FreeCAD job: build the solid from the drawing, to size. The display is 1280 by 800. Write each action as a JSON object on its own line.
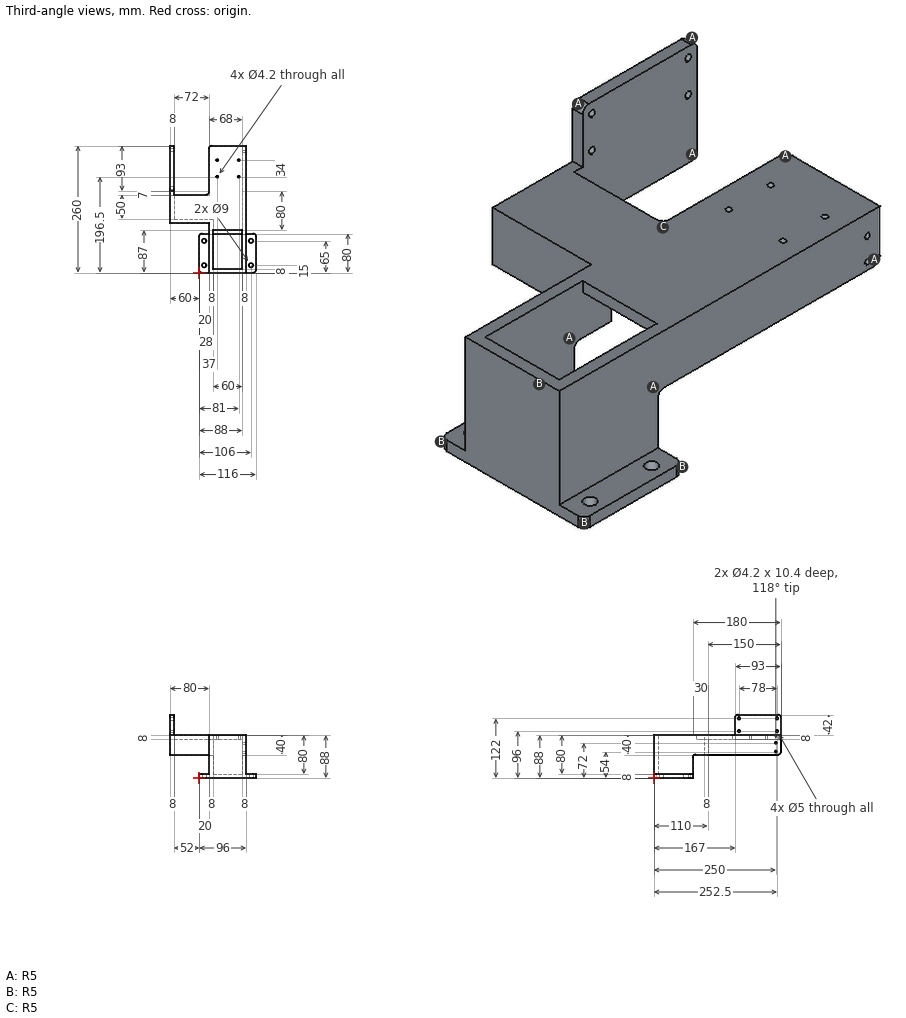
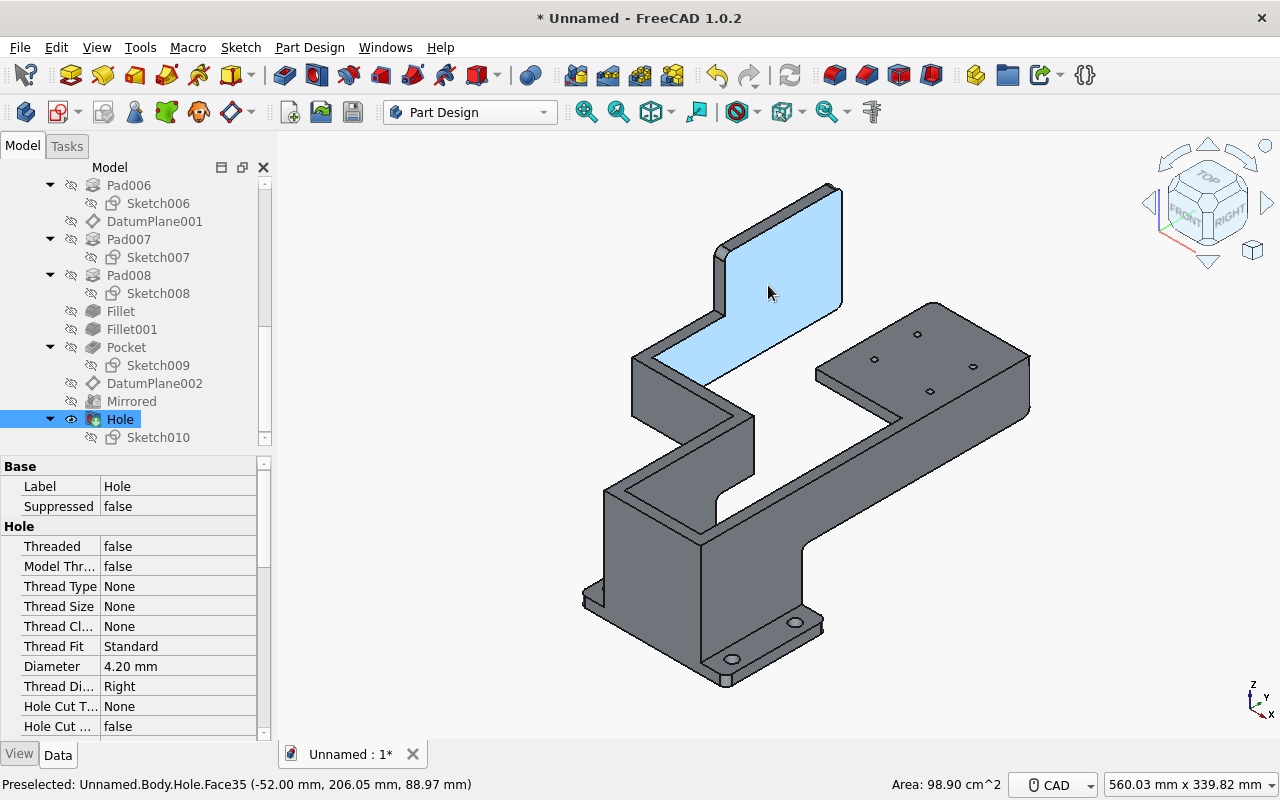
{"action": "left_click", "coordinate": [58, 112]}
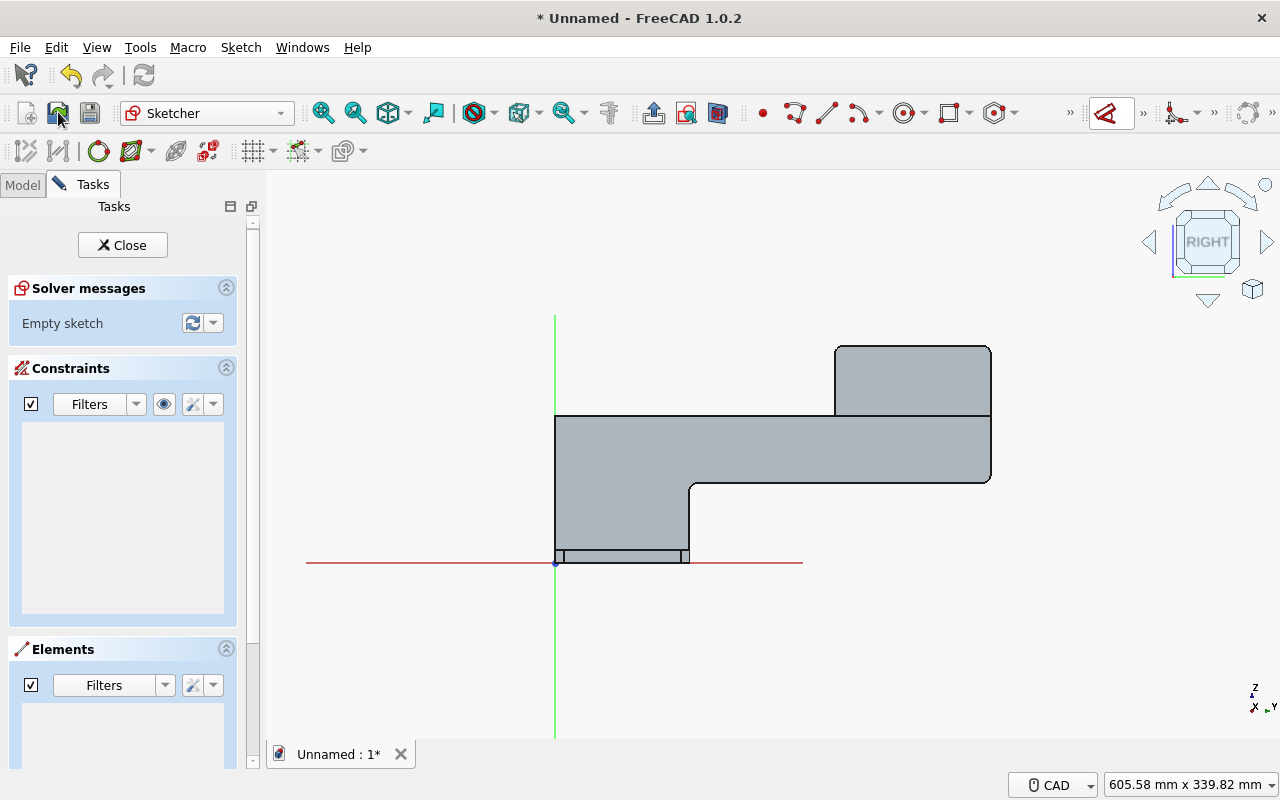
{"action": "left_click", "coordinate": [718, 114]}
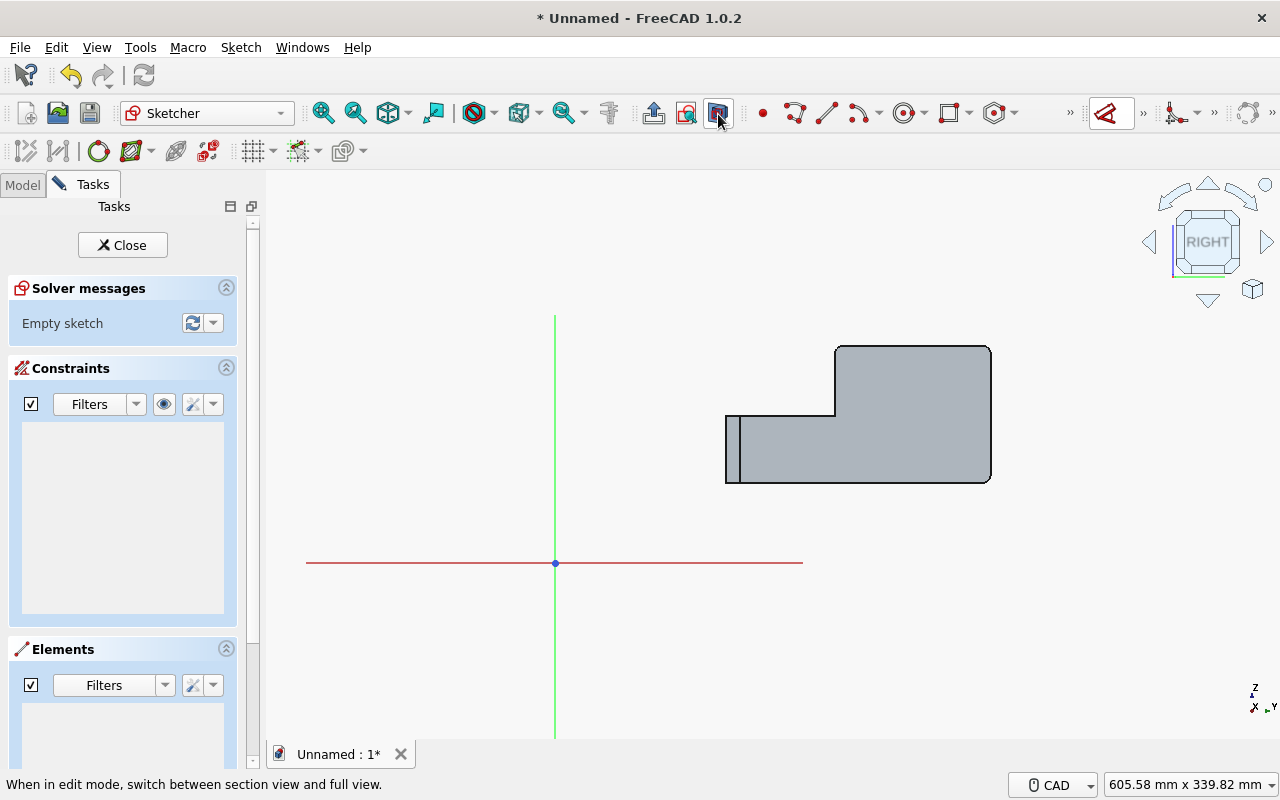
{"action": "scroll", "coordinate": [981, 357], "scroll_direction": "up", "scroll_amount": 7}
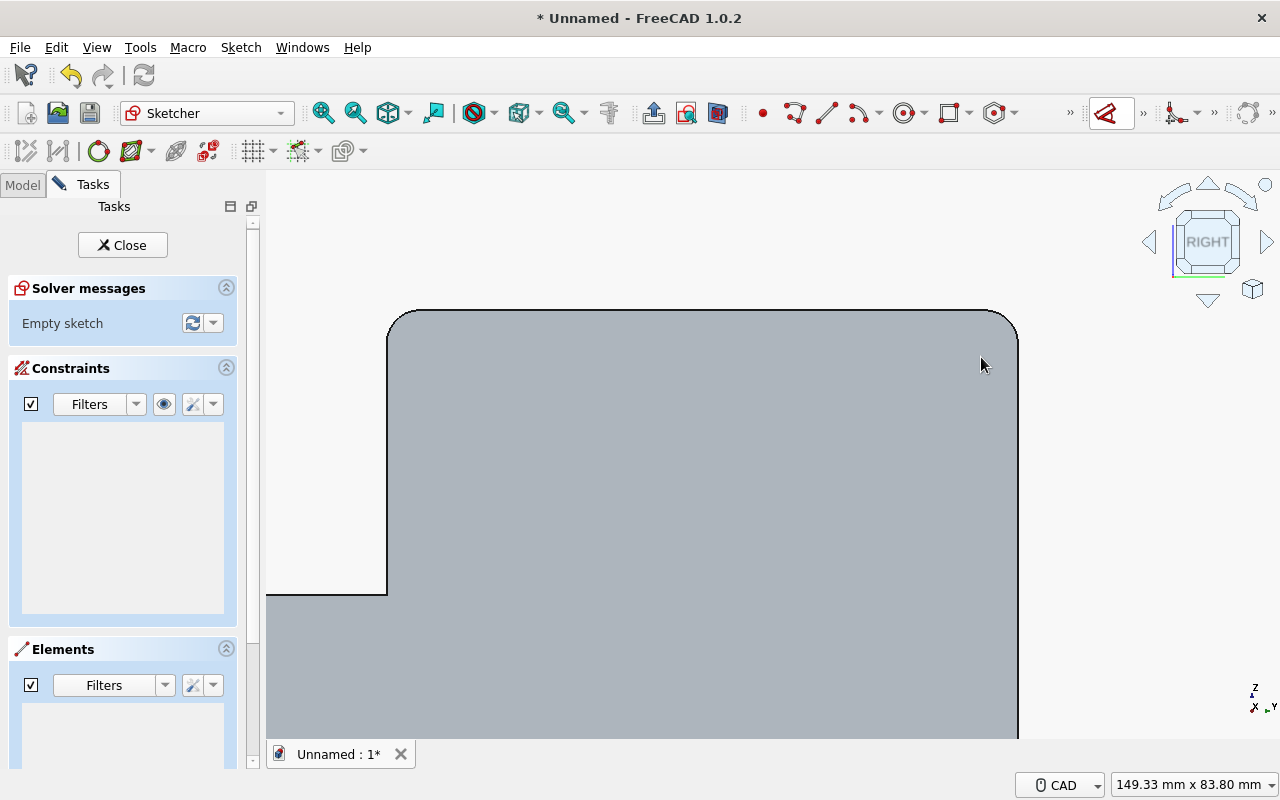
{"action": "left_click", "coordinate": [904, 114]}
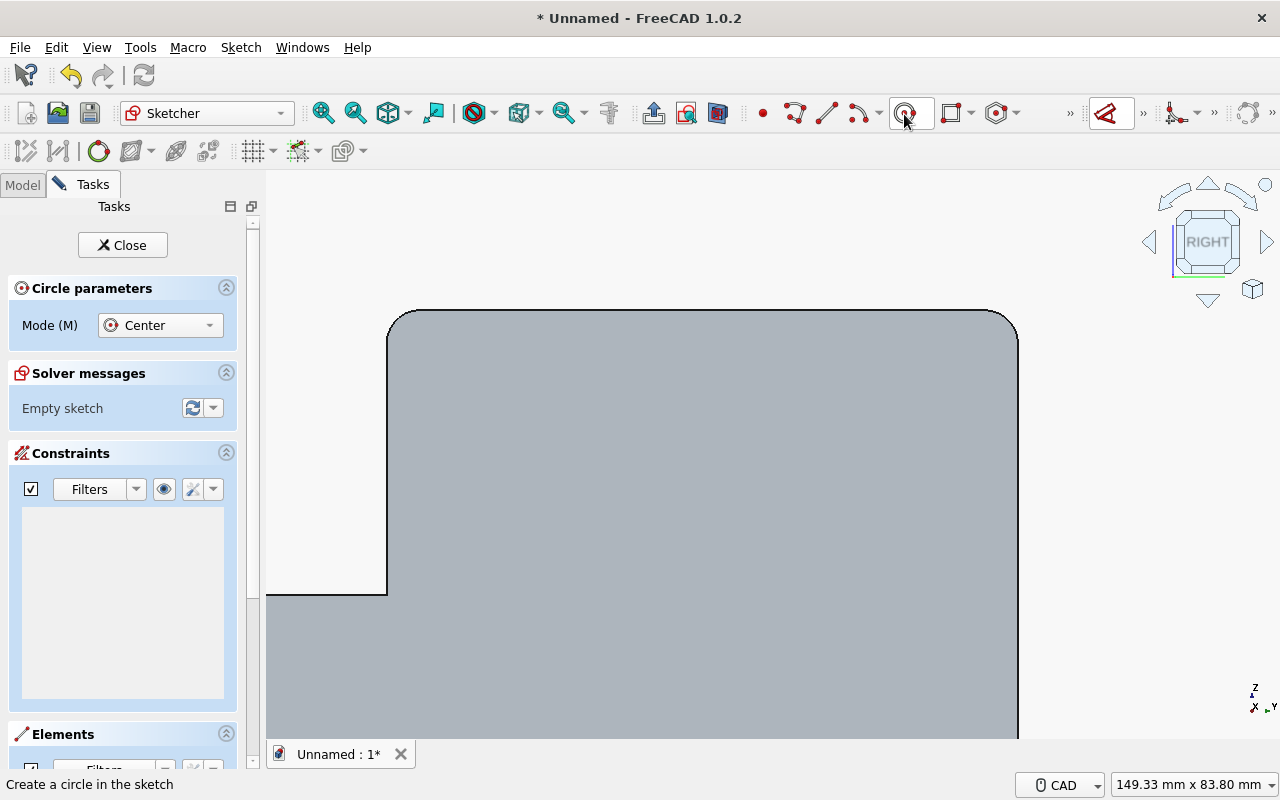
{"action": "scroll", "coordinate": [967, 541], "scroll_direction": "up", "scroll_amount": 2}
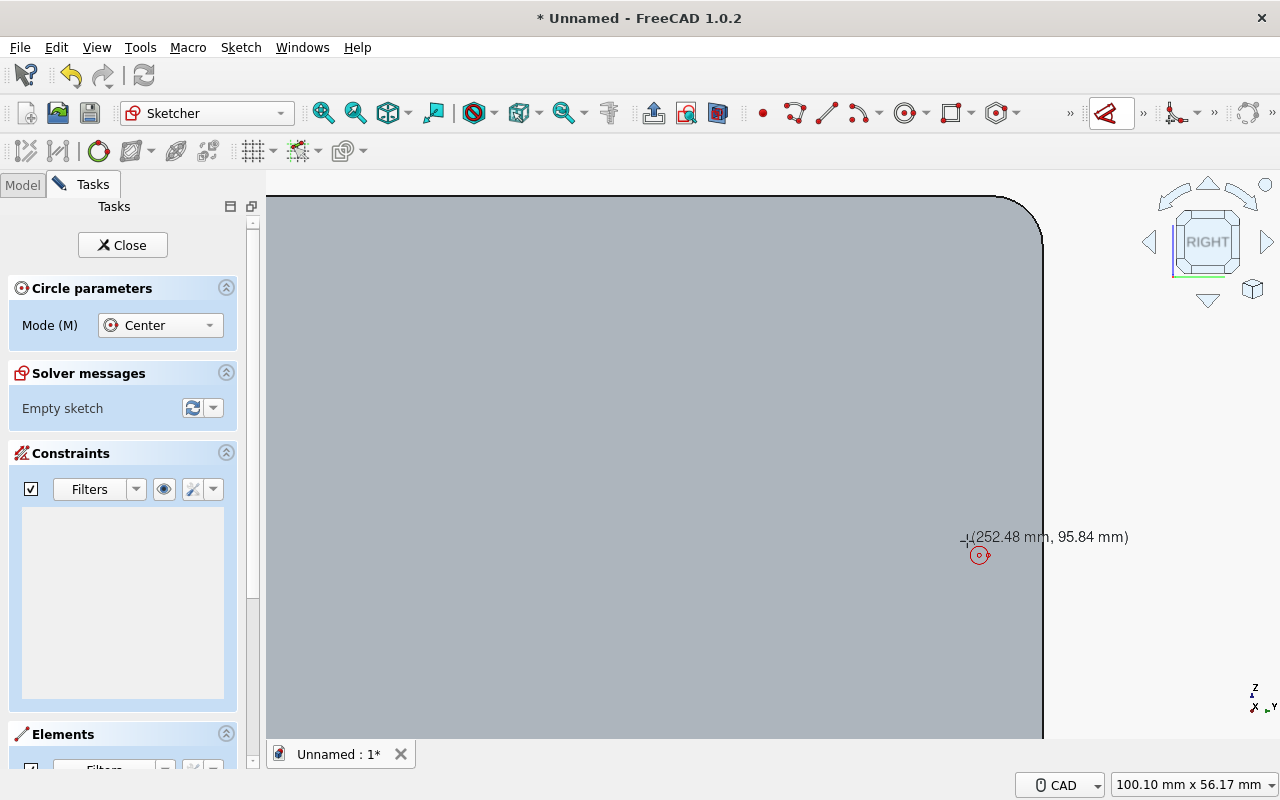
{"action": "left_click", "coordinate": [967, 541]}
{"action": "left_click", "coordinate": [985, 523]}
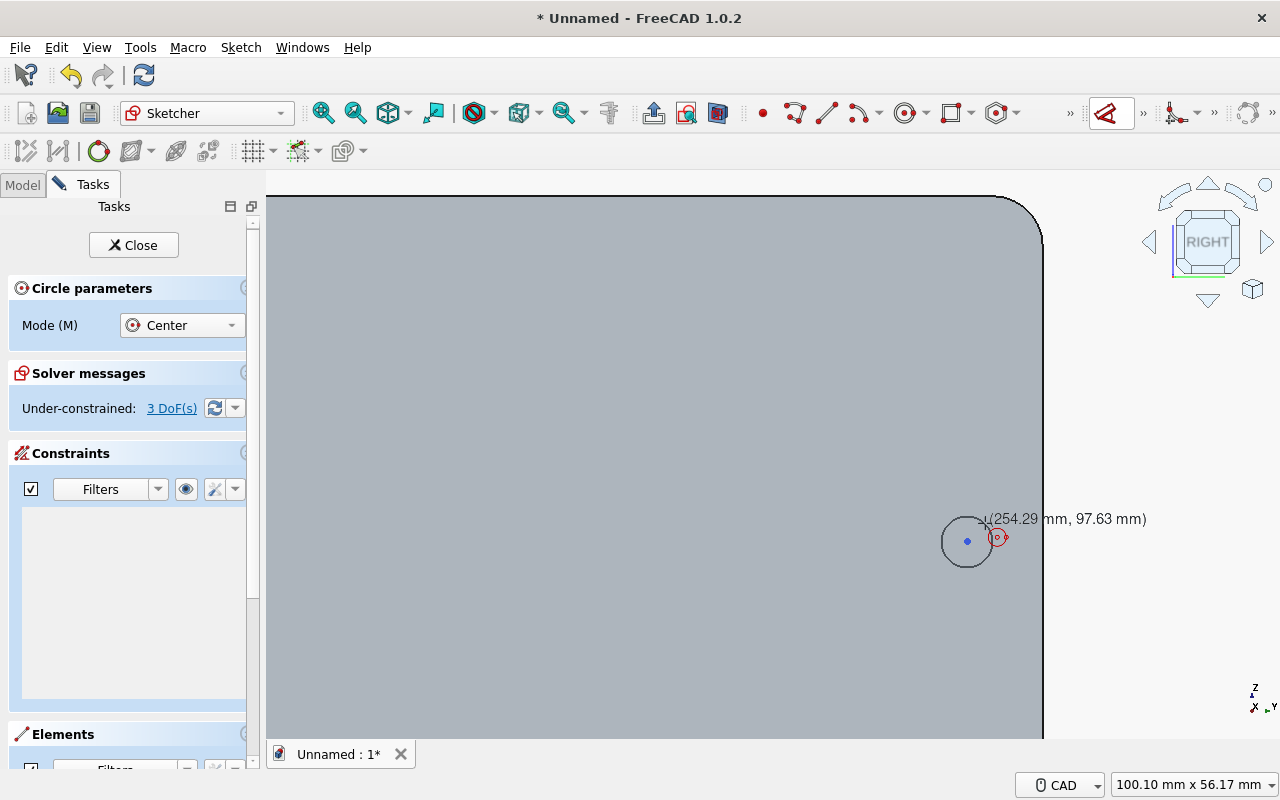
{"action": "left_click", "coordinate": [967, 277]}
{"action": "left_click", "coordinate": [985, 259]}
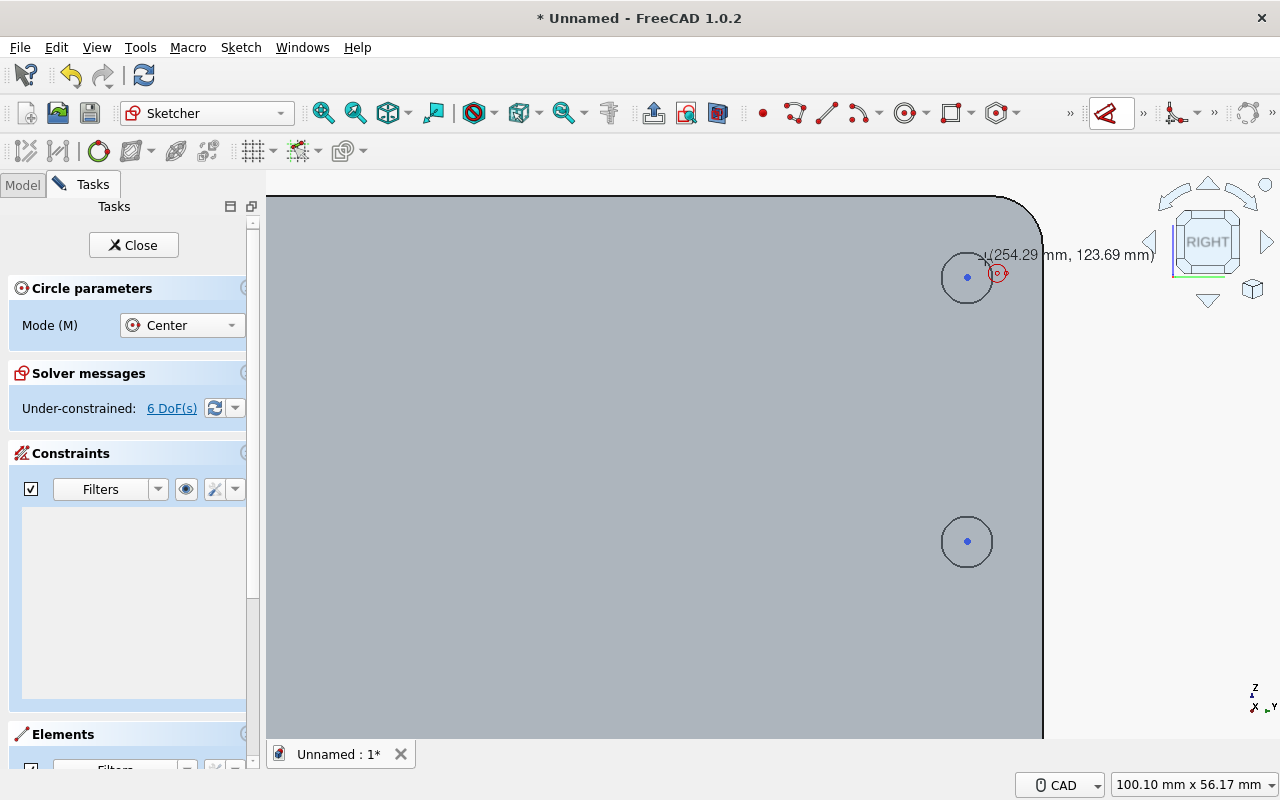
{"action": "scroll", "coordinate": [974, 547], "scroll_direction": "down", "scroll_amount": 2}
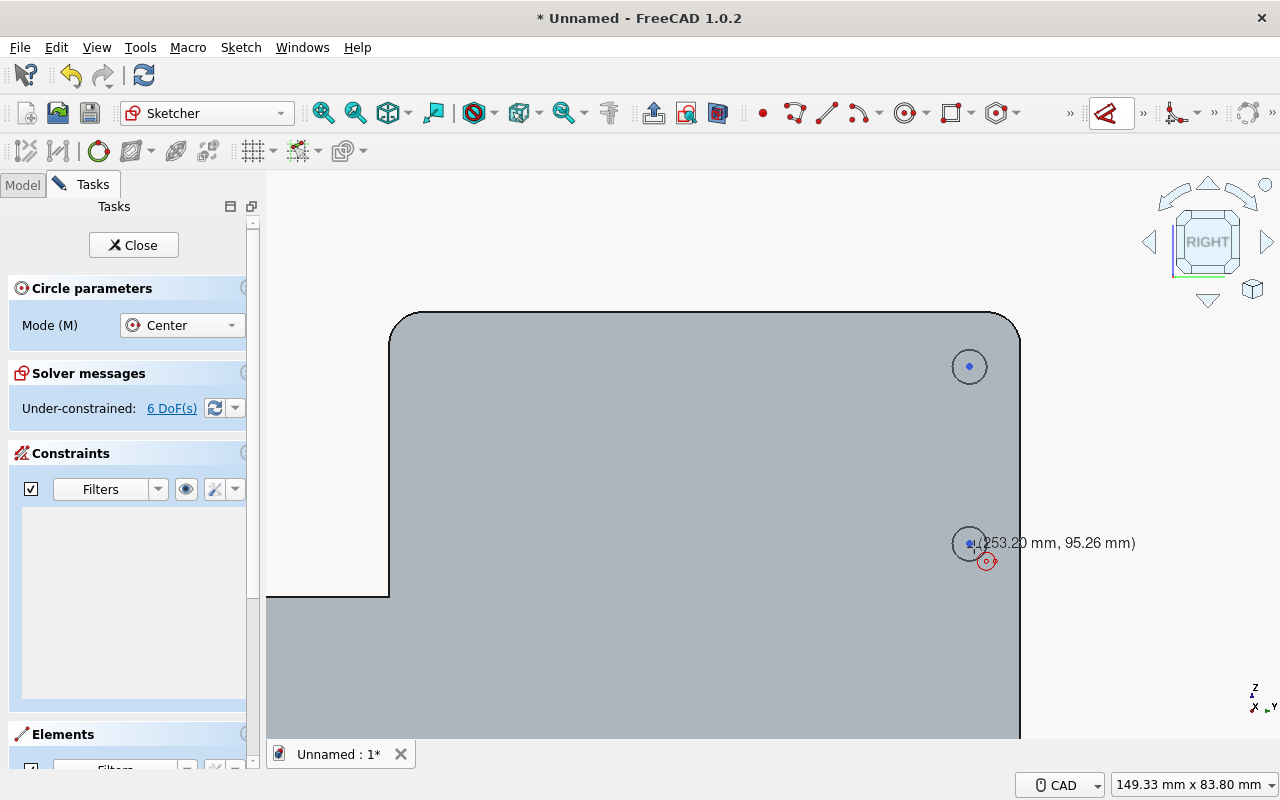
{"action": "scroll", "coordinate": [440, 366], "scroll_direction": "up", "scroll_amount": 2}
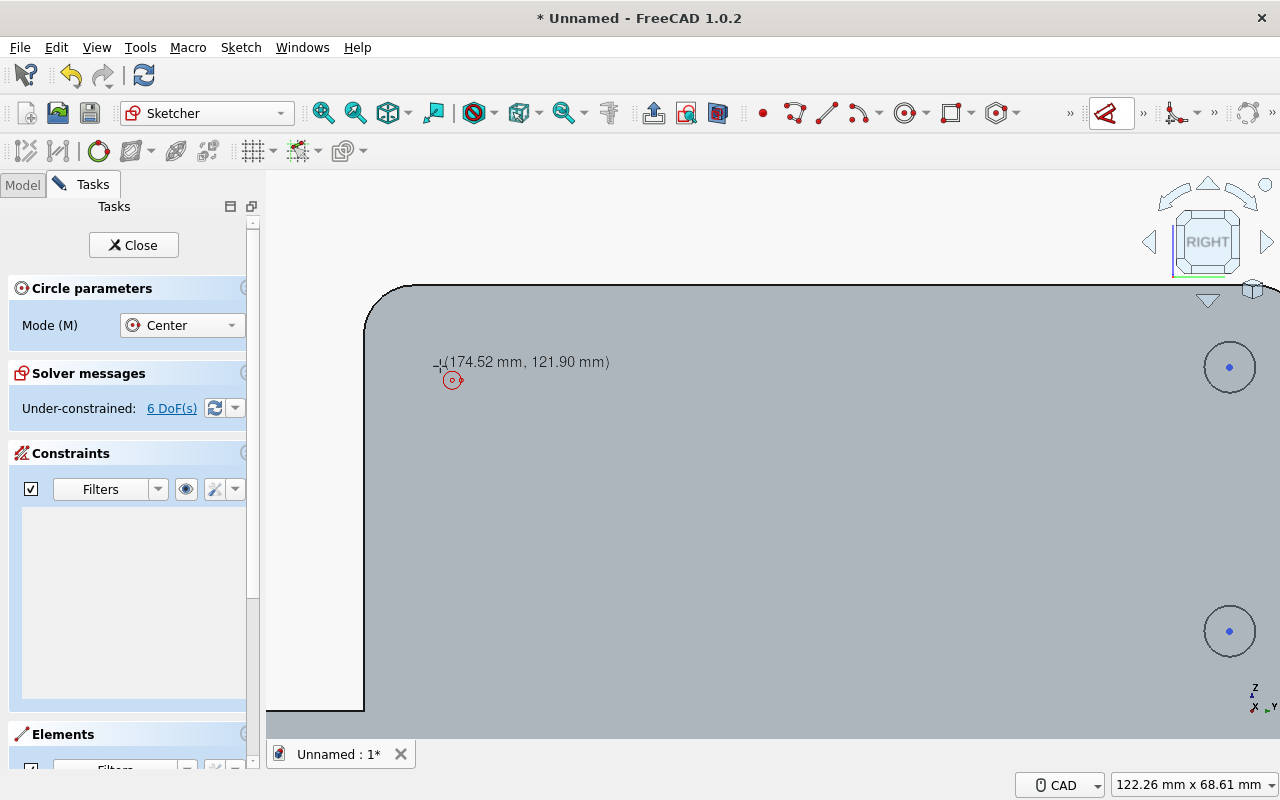
{"action": "left_click", "coordinate": [440, 366]}
{"action": "left_click", "coordinate": [458, 348]}